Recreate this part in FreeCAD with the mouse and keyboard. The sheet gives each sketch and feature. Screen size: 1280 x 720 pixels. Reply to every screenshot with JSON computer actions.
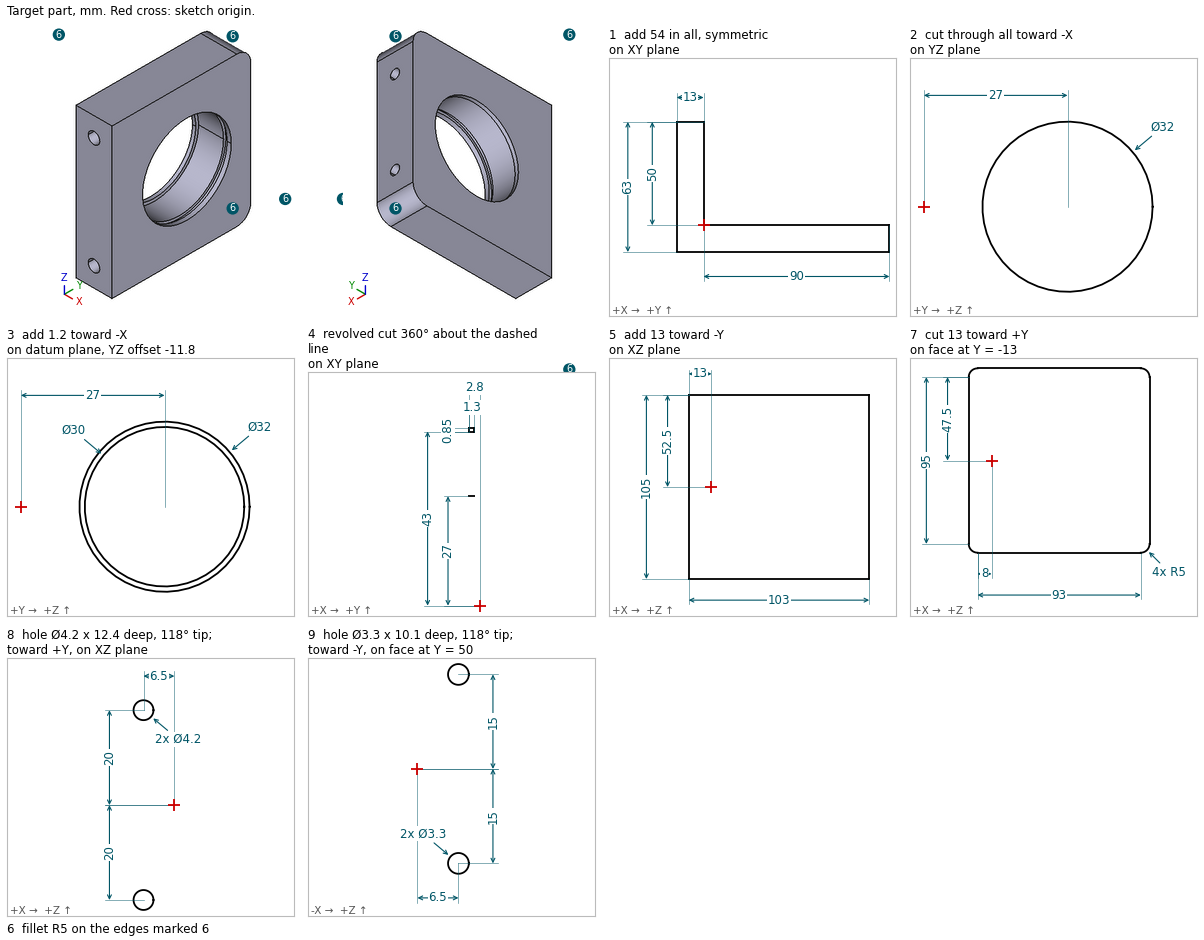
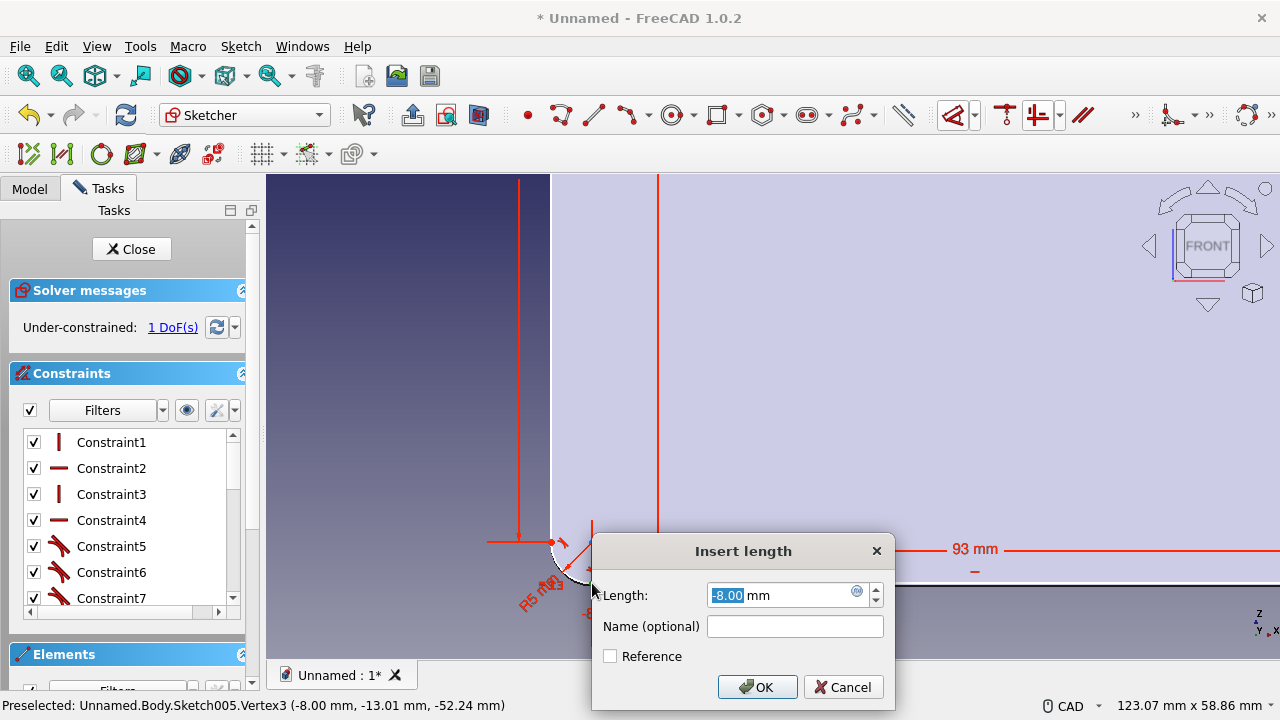
{"action": "type", "text": "-8"}
{"action": "key", "text": "Return"}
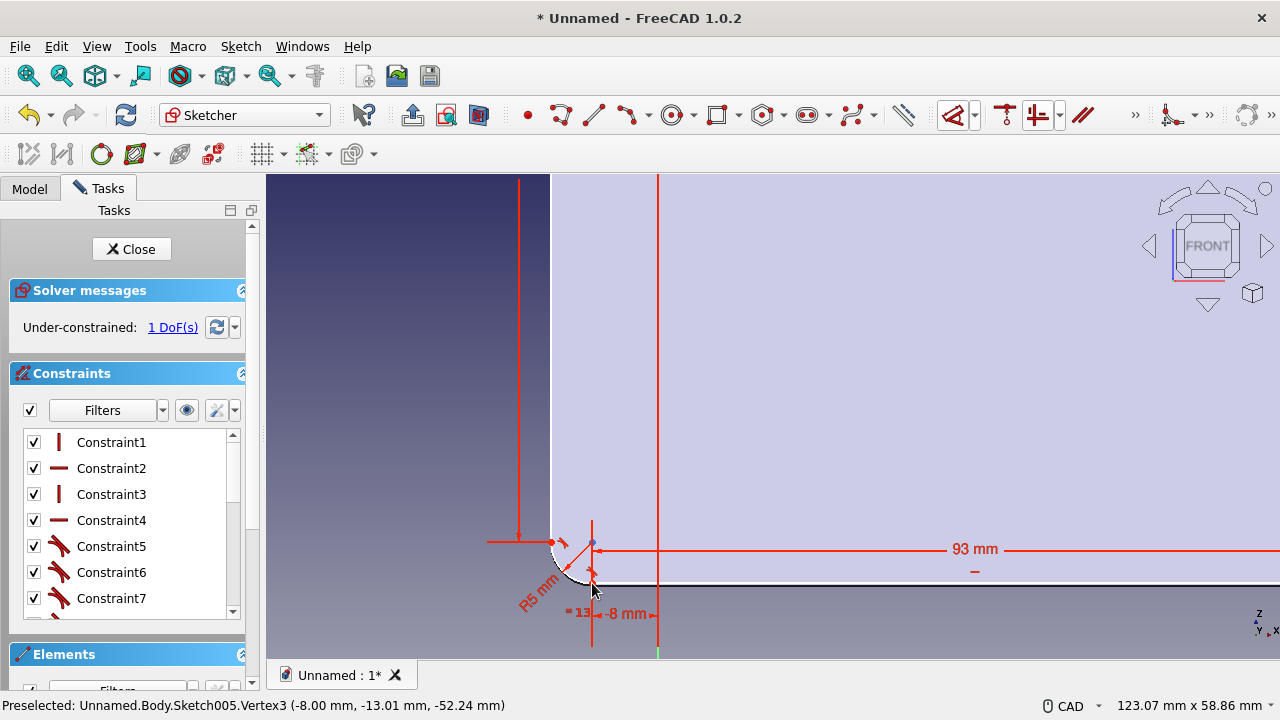
{"action": "scroll", "coordinate": [547, 570], "scroll_direction": "down", "scroll_amount": 5}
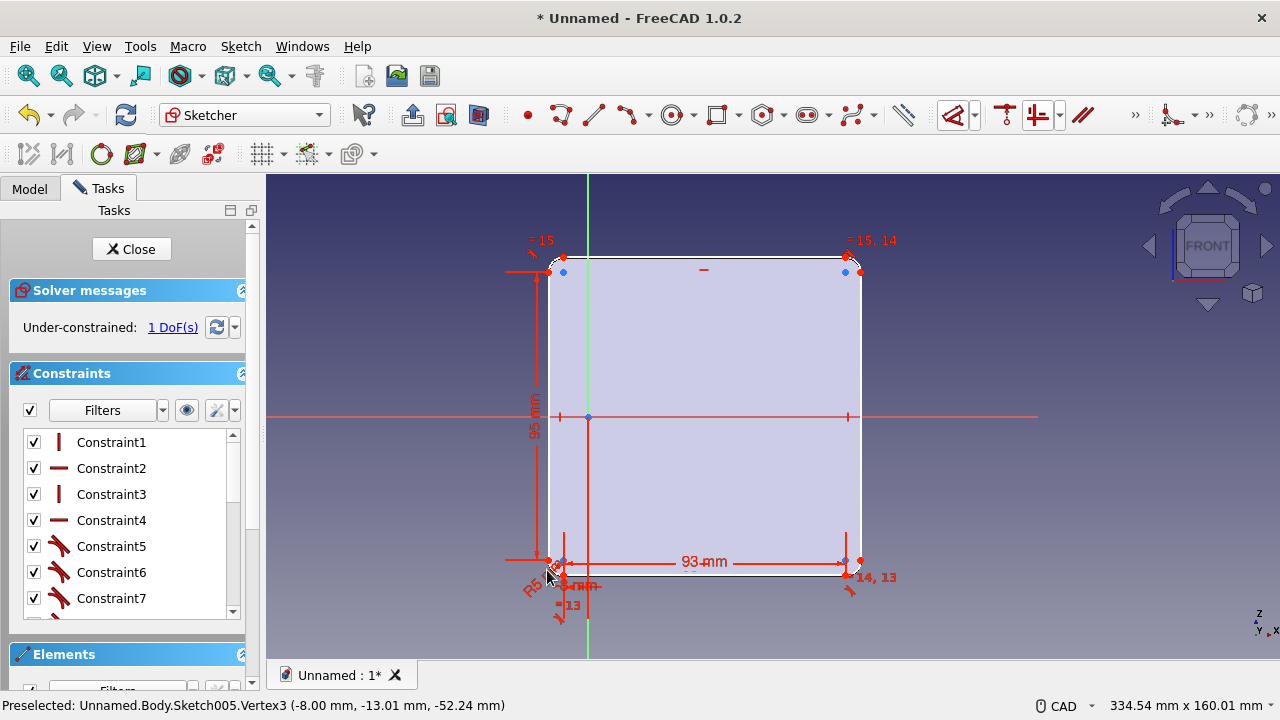
{"action": "left_click", "coordinate": [549, 272]}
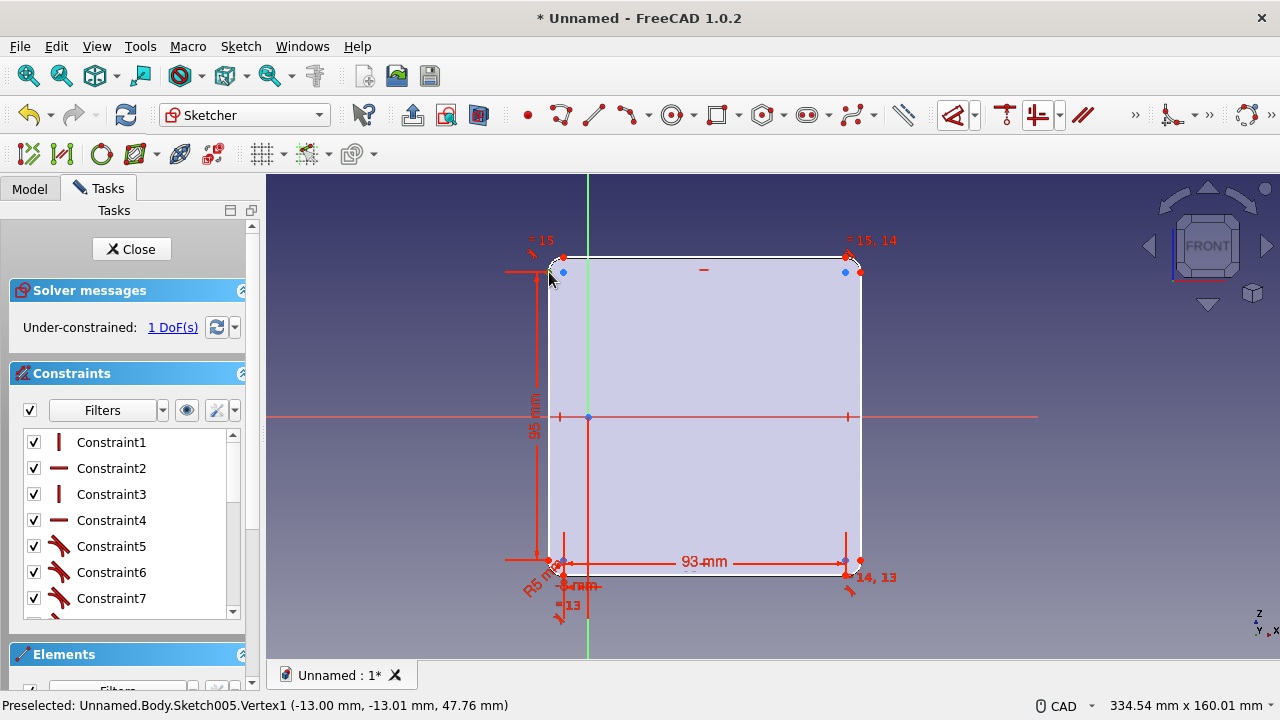
{"action": "key", "text": "i"}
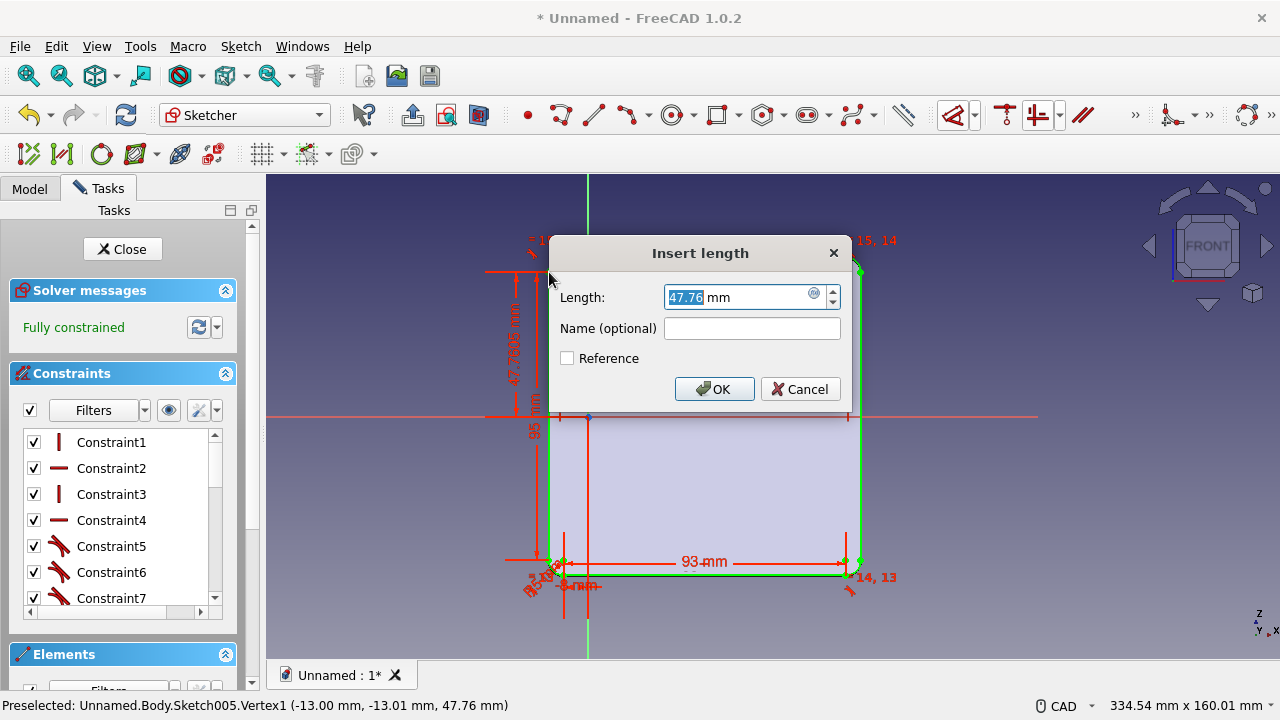
{"action": "type", "text": "47.5"}
{"action": "key", "text": "Return"}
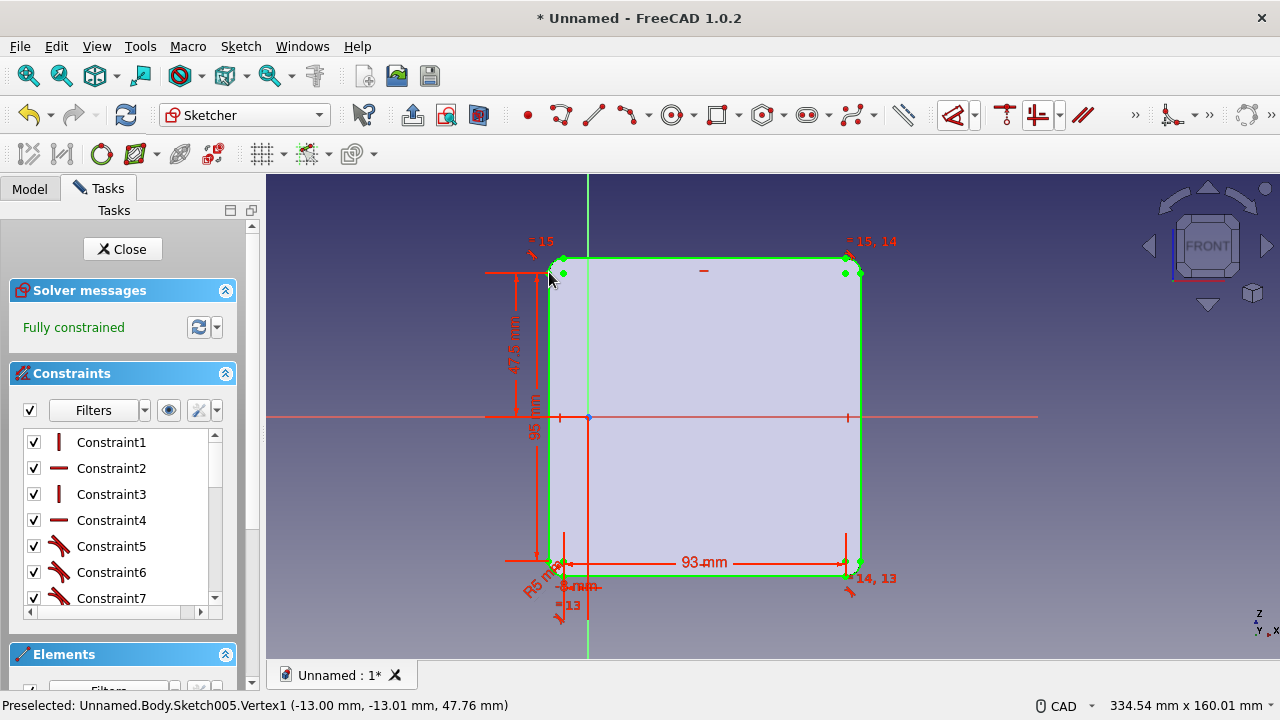
{"action": "left_click", "coordinate": [123, 249]}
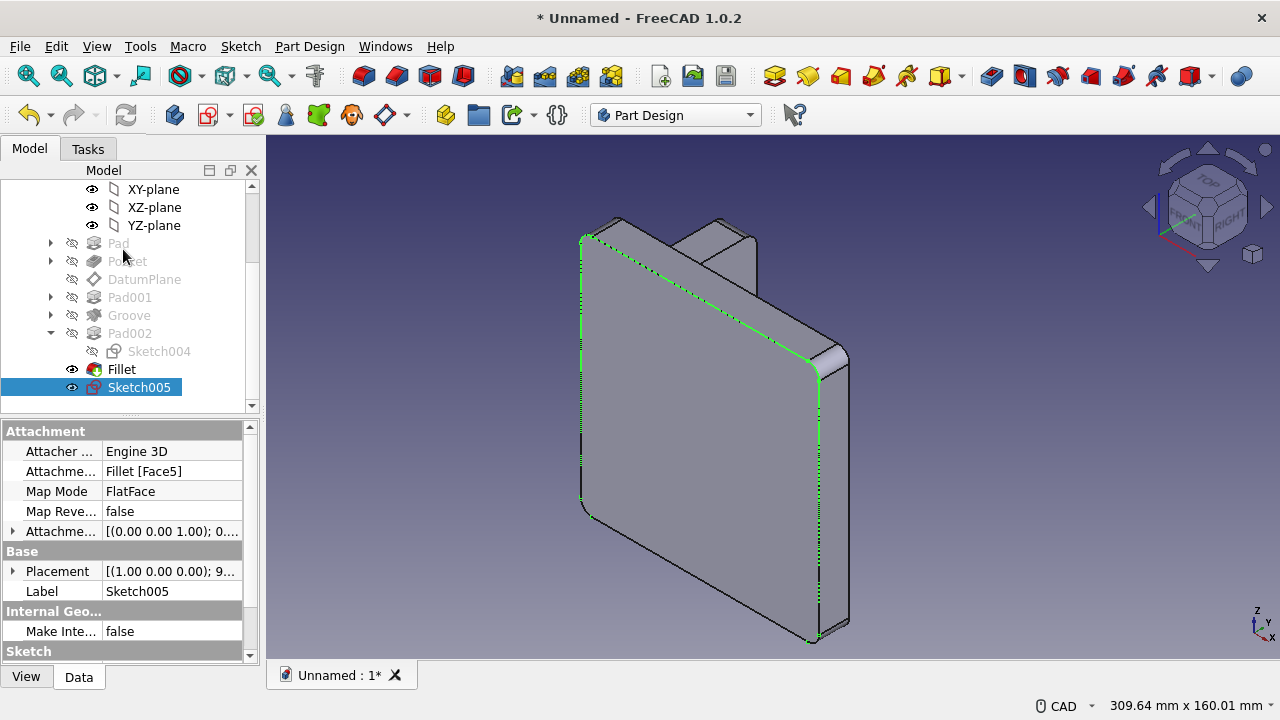
{"action": "left_click", "coordinate": [992, 76]}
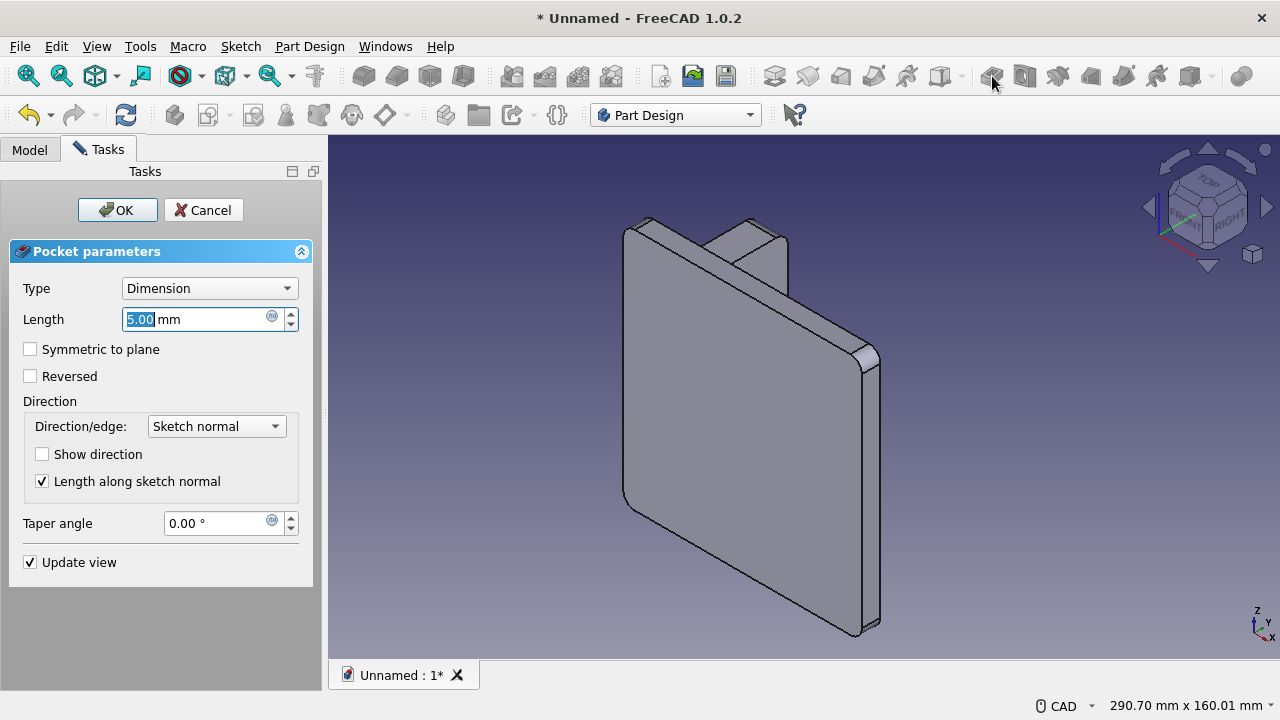
{"action": "type", "text": "13"}
{"action": "key", "text": "Tab"}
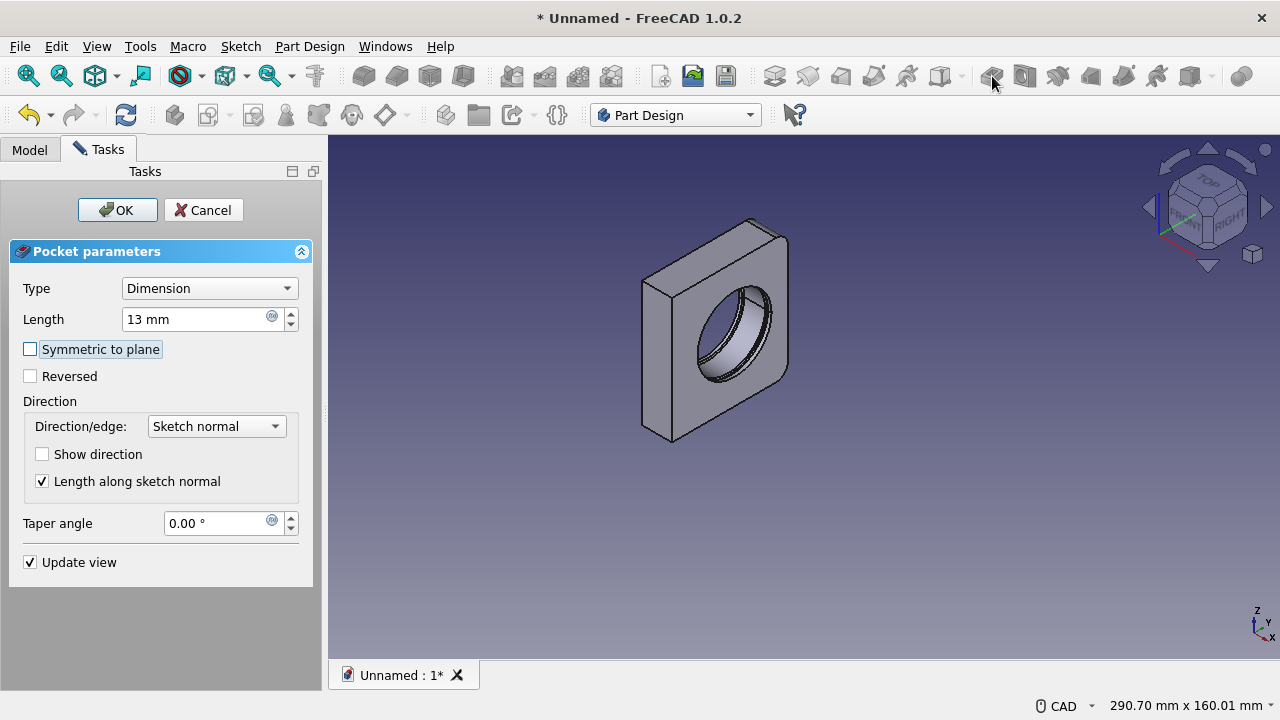
{"action": "left_click", "coordinate": [118, 210]}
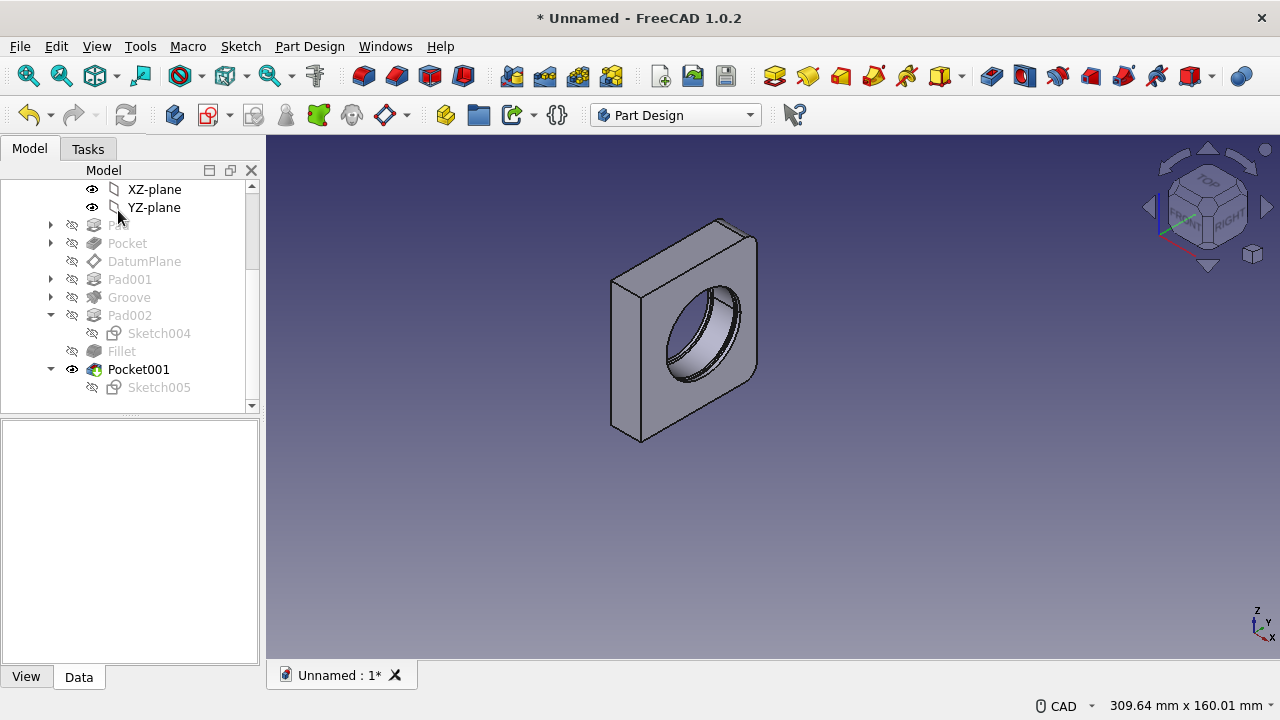
{"action": "left_click", "coordinate": [29, 76]}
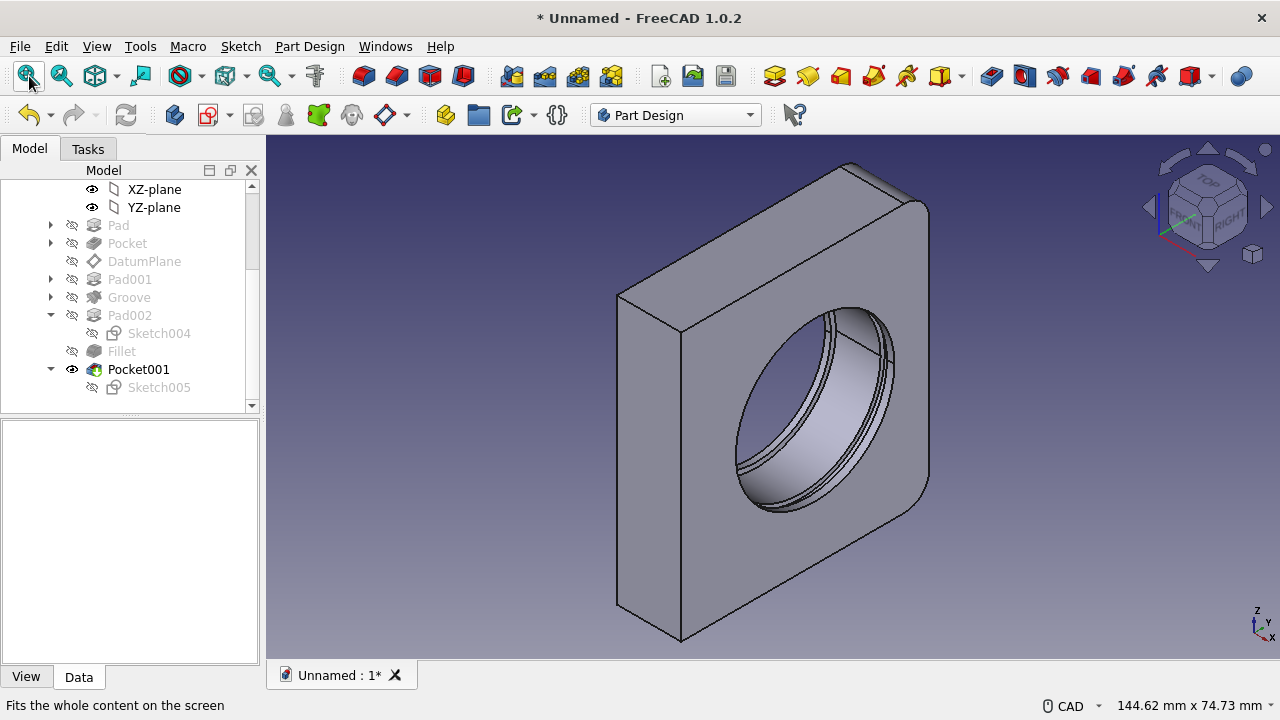
{"action": "left_click", "coordinate": [208, 116]}